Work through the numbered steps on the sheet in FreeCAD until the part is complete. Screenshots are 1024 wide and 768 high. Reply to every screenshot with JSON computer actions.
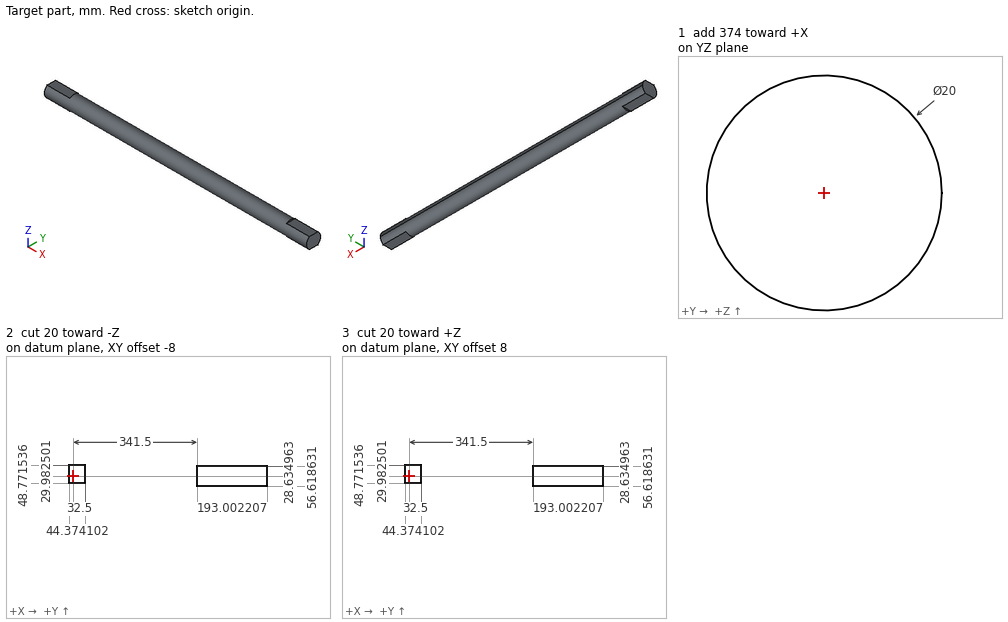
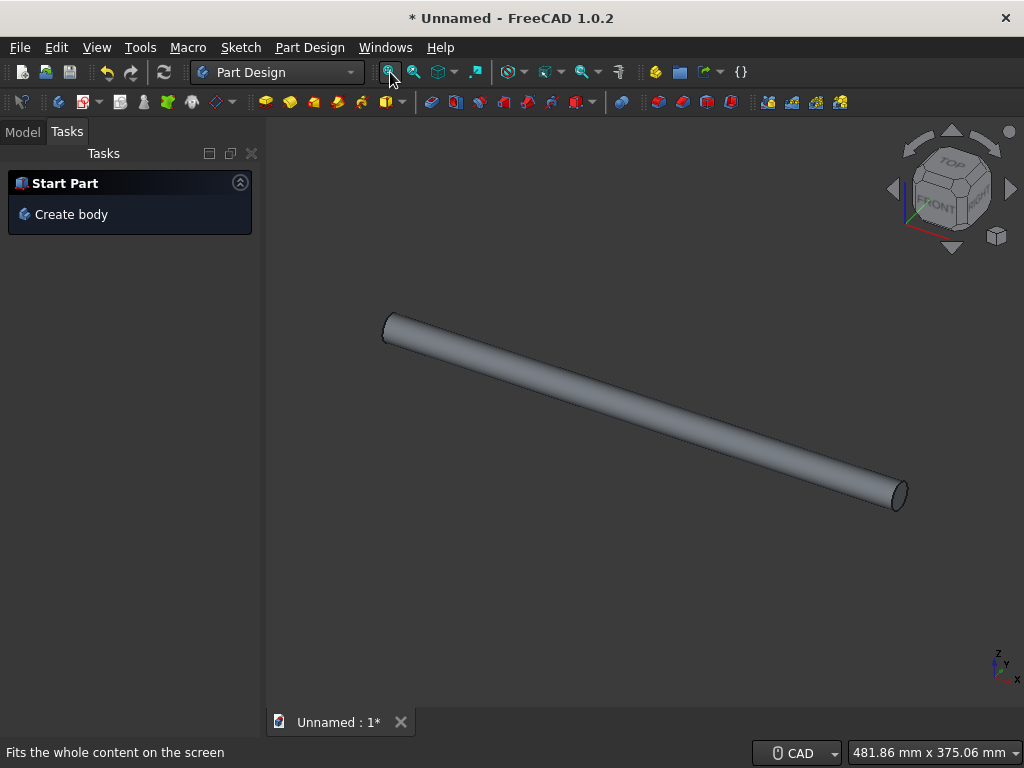
{"action": "left_click", "coordinate": [23, 131]}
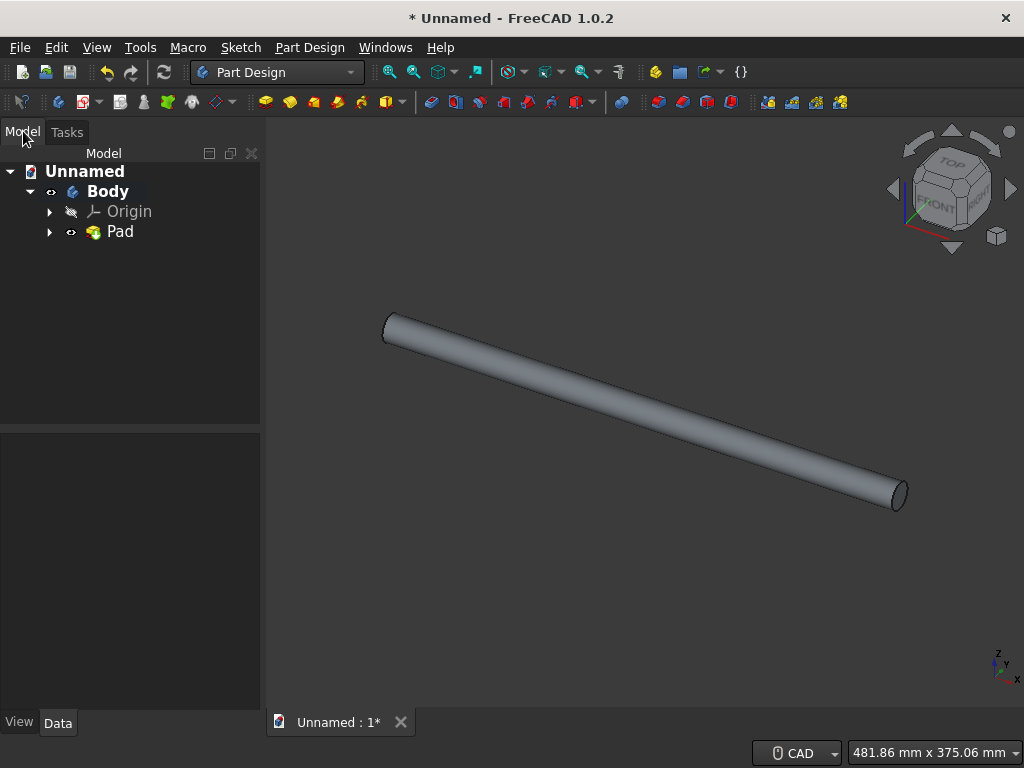
{"action": "left_click", "coordinate": [50, 212]}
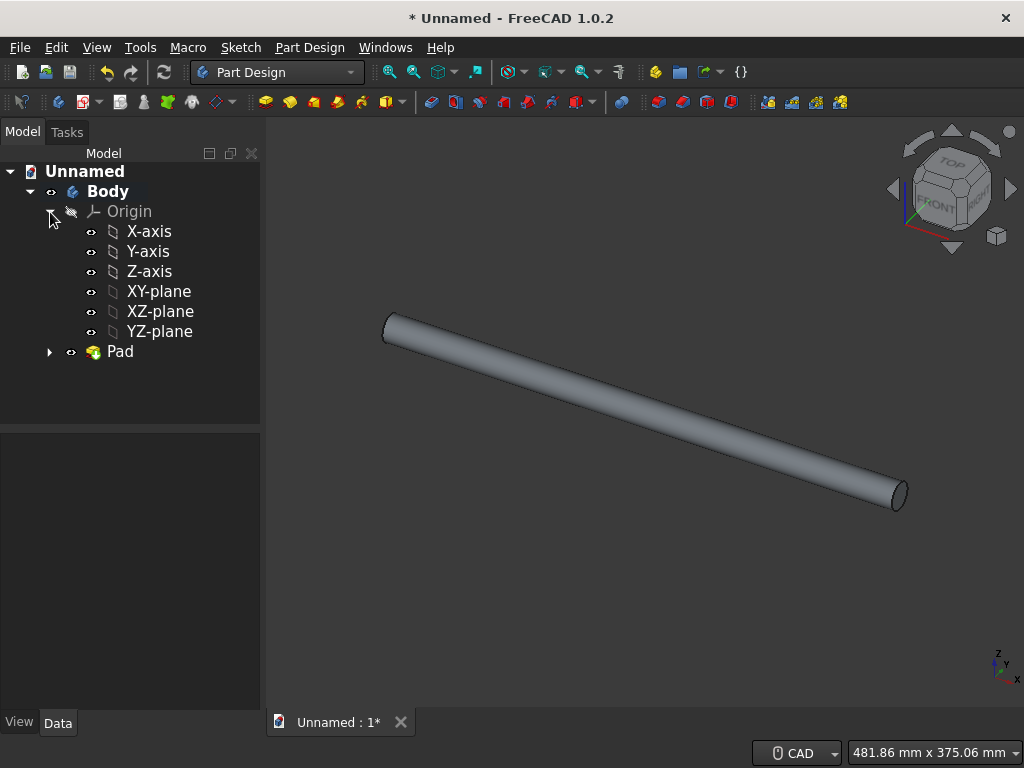
{"action": "left_click", "coordinate": [136, 292]}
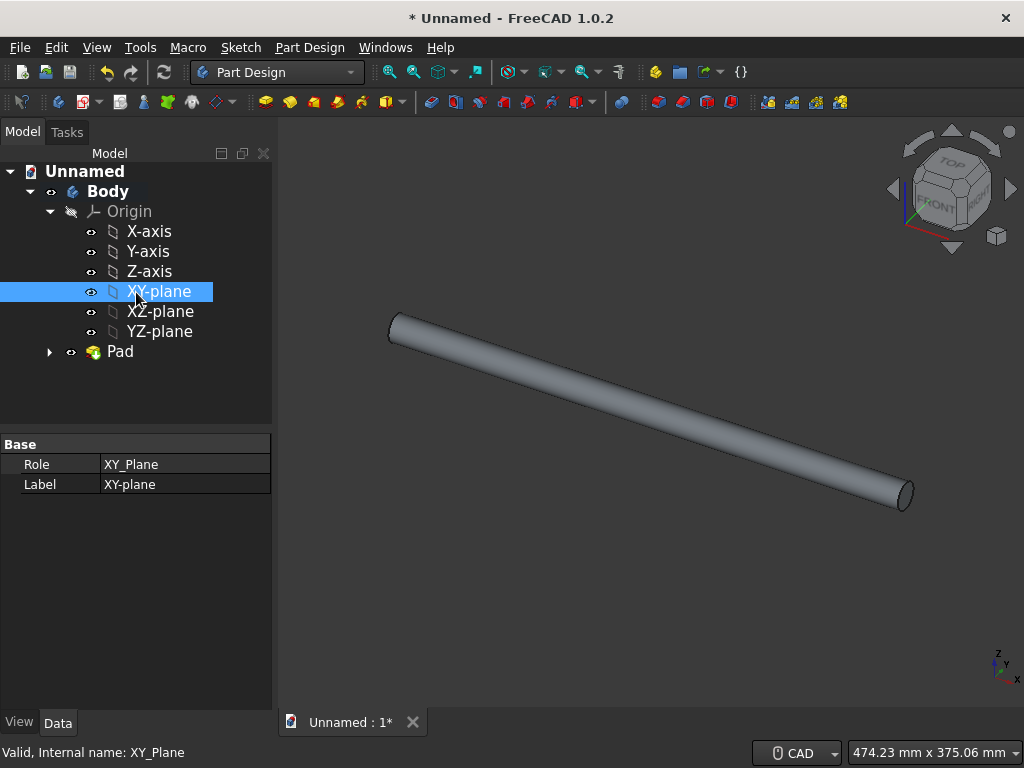
{"action": "left_click", "coordinate": [216, 102]}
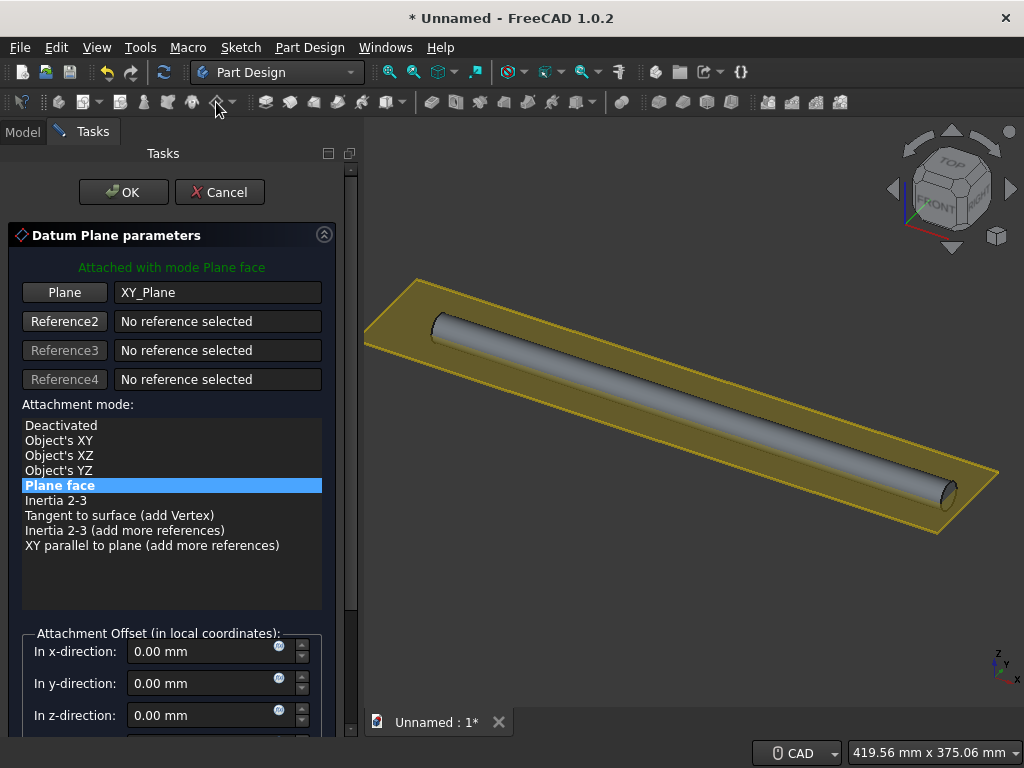
{"action": "triple_click", "coordinate": [210, 715]}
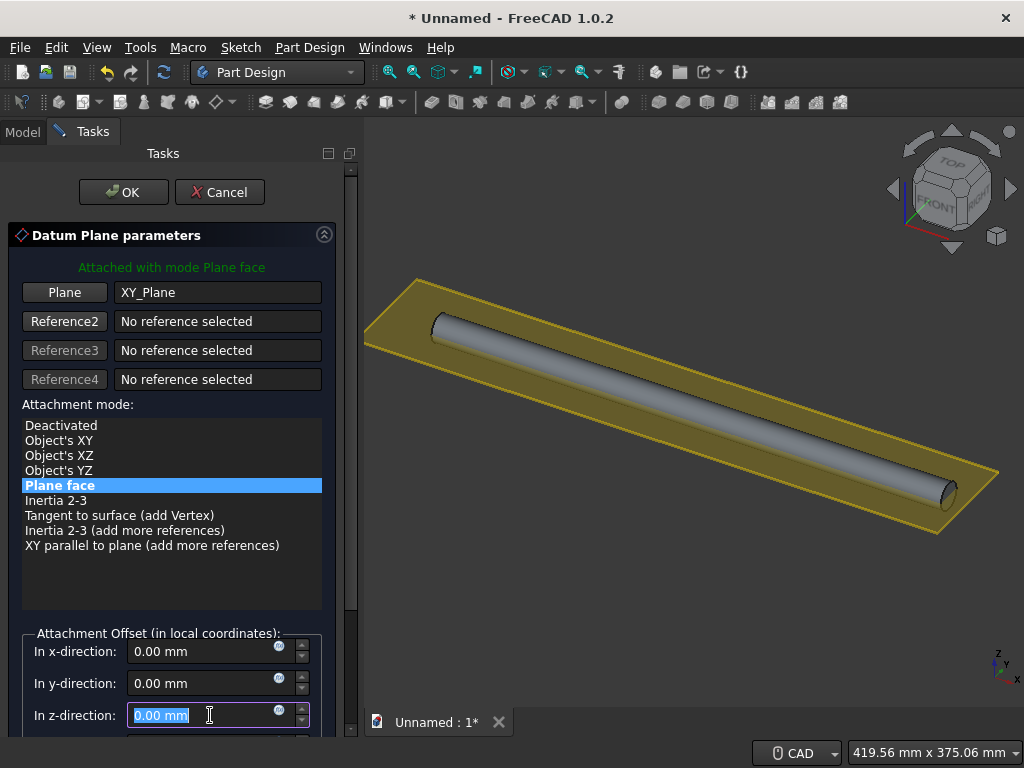
{"action": "type", "text": "-8"}
{"action": "key", "text": "Tab"}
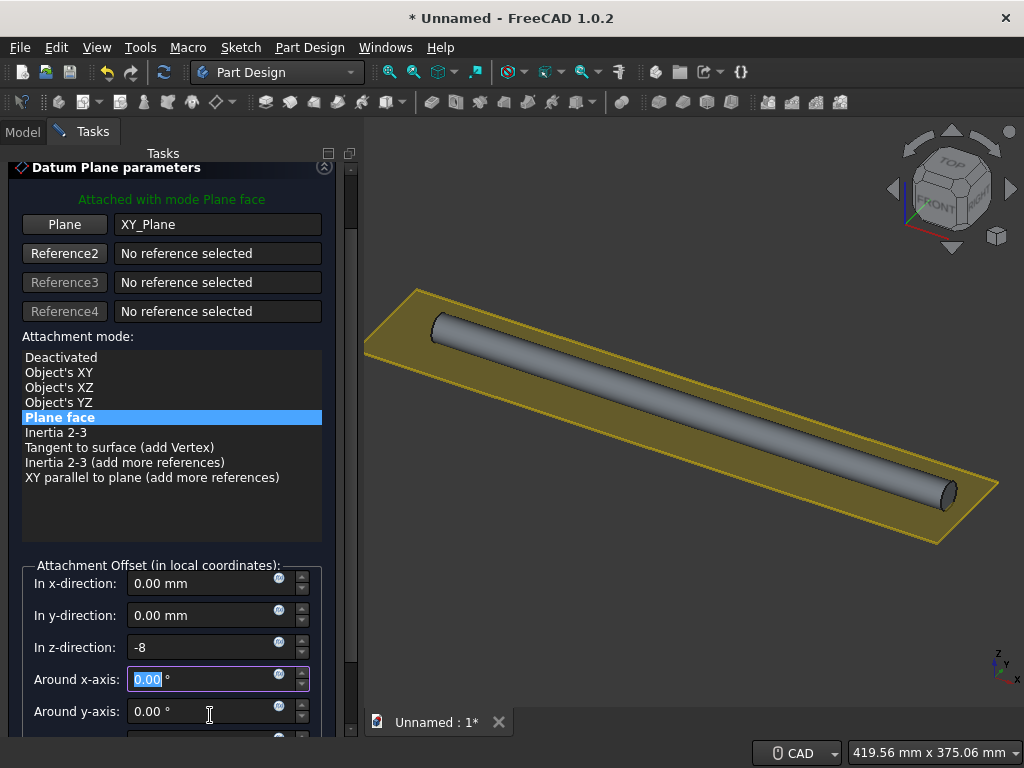
{"action": "scroll", "coordinate": [351, 450], "scroll_direction": "up", "scroll_amount": 2}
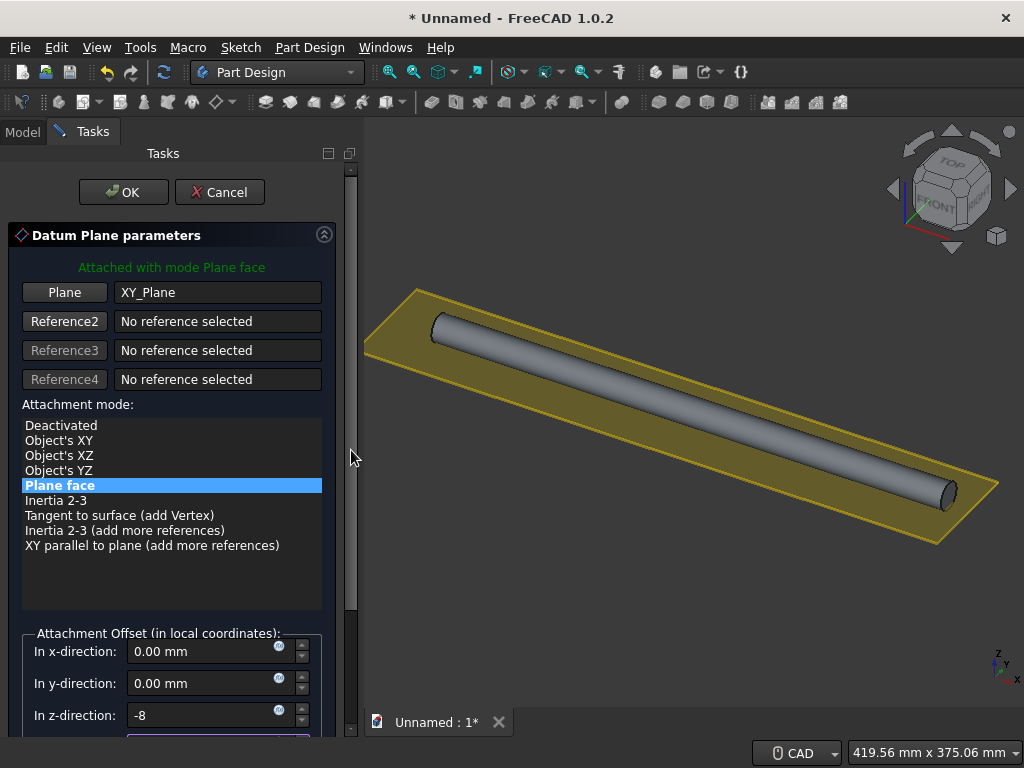
{"action": "left_click", "coordinate": [124, 192]}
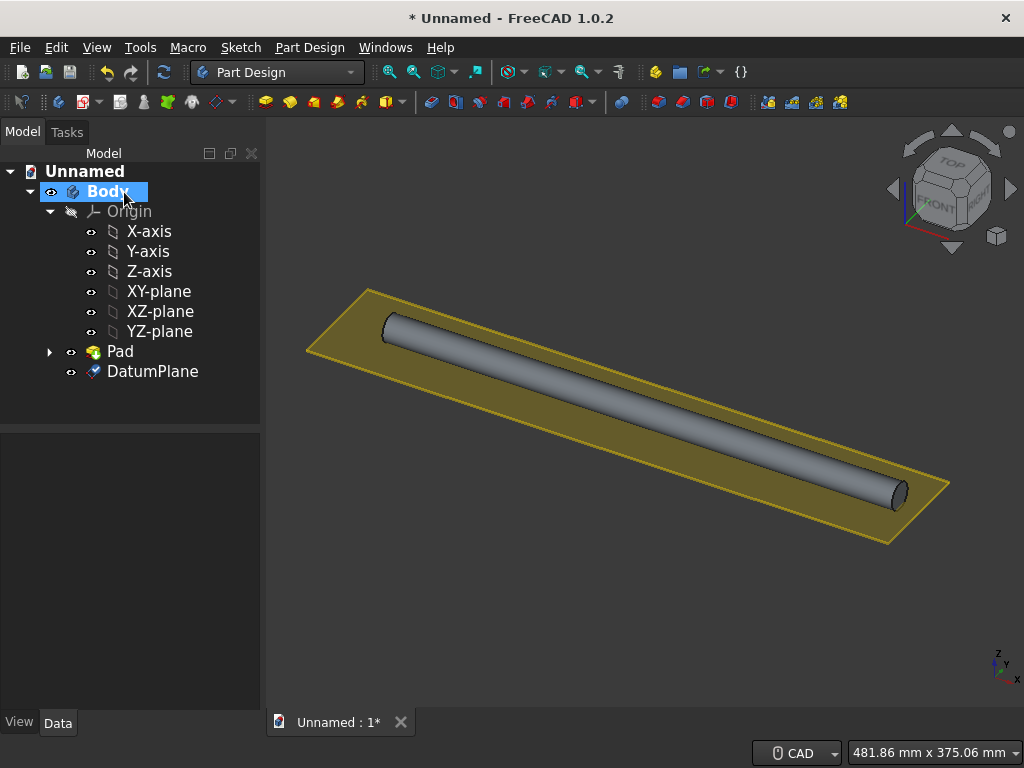
{"action": "left_click", "coordinate": [116, 372]}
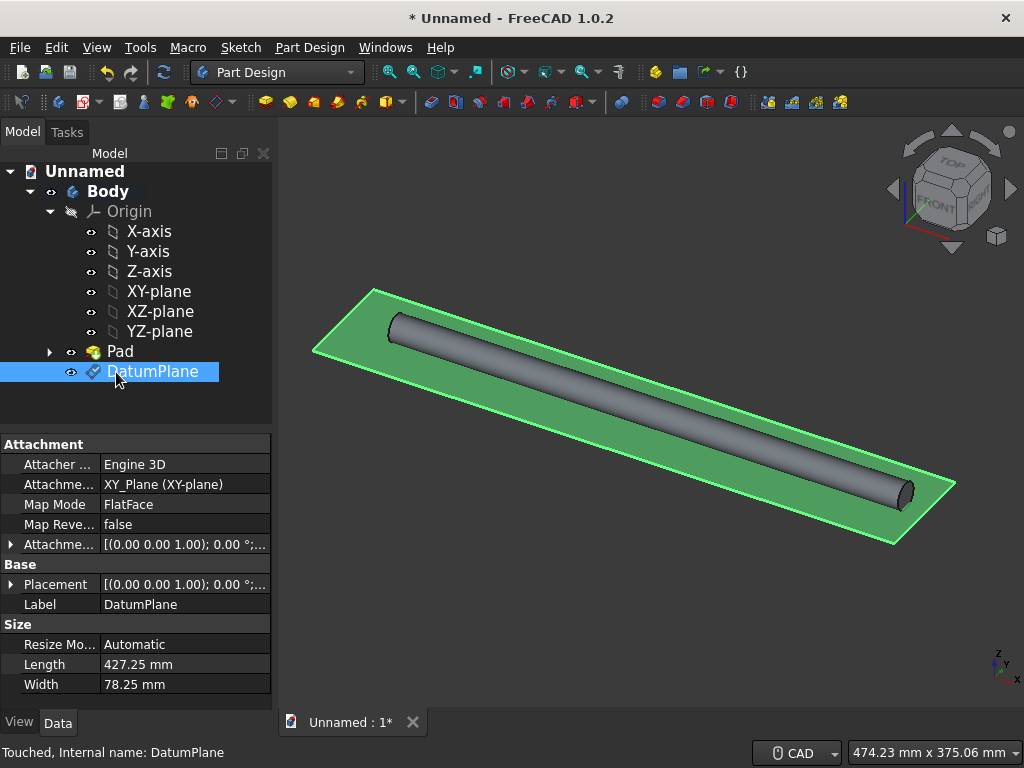
{"action": "left_click", "coordinate": [84, 102]}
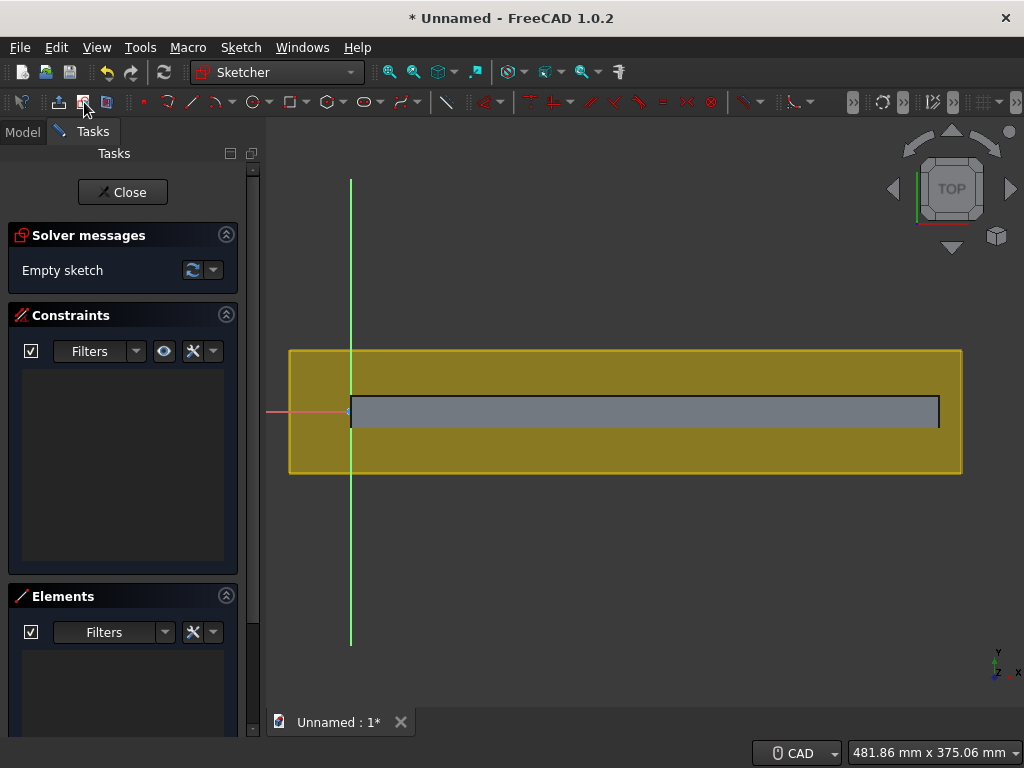
{"action": "left_click", "coordinate": [108, 102]}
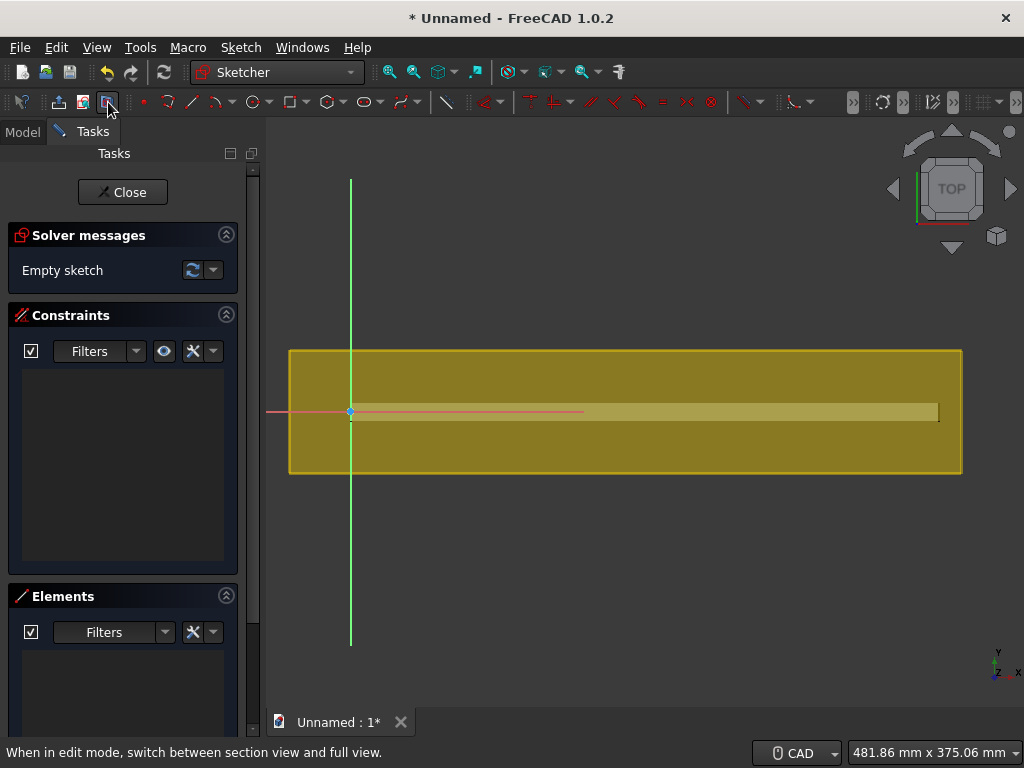
{"action": "scroll", "coordinate": [425, 413], "scroll_direction": "down", "scroll_amount": 4}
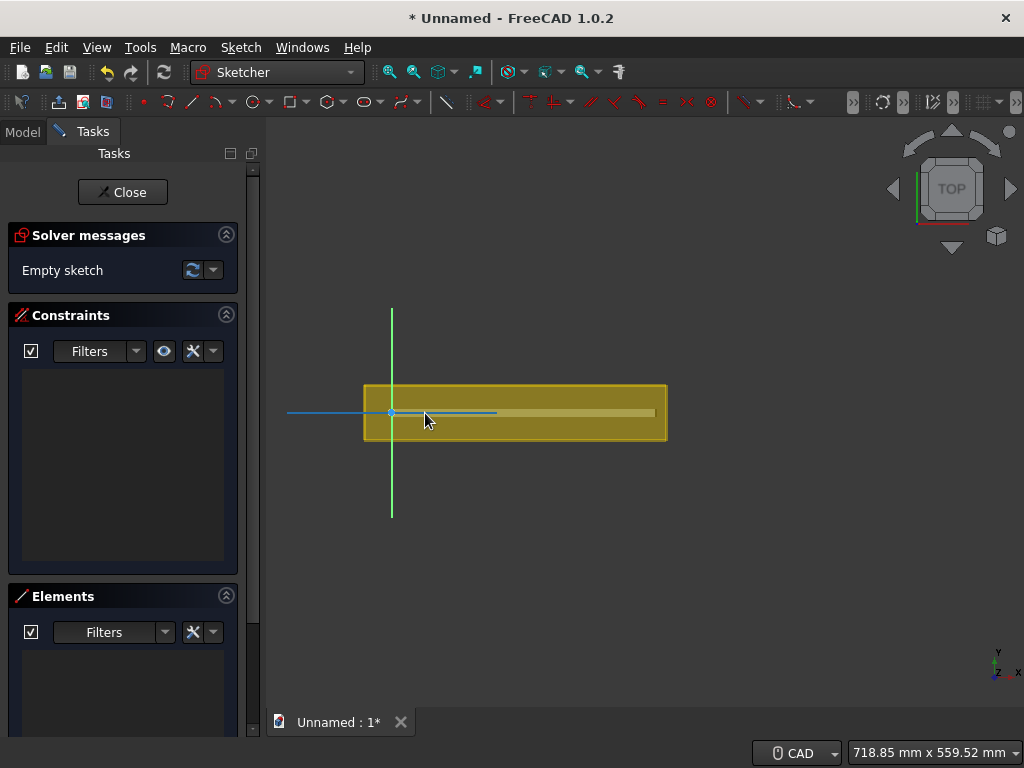
{"action": "left_click", "coordinate": [290, 102]}